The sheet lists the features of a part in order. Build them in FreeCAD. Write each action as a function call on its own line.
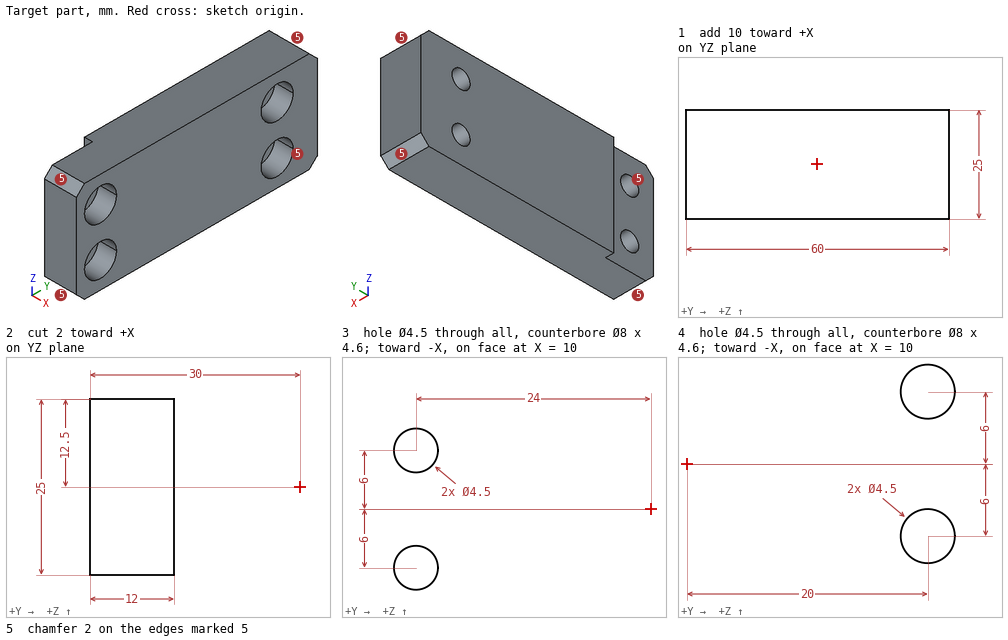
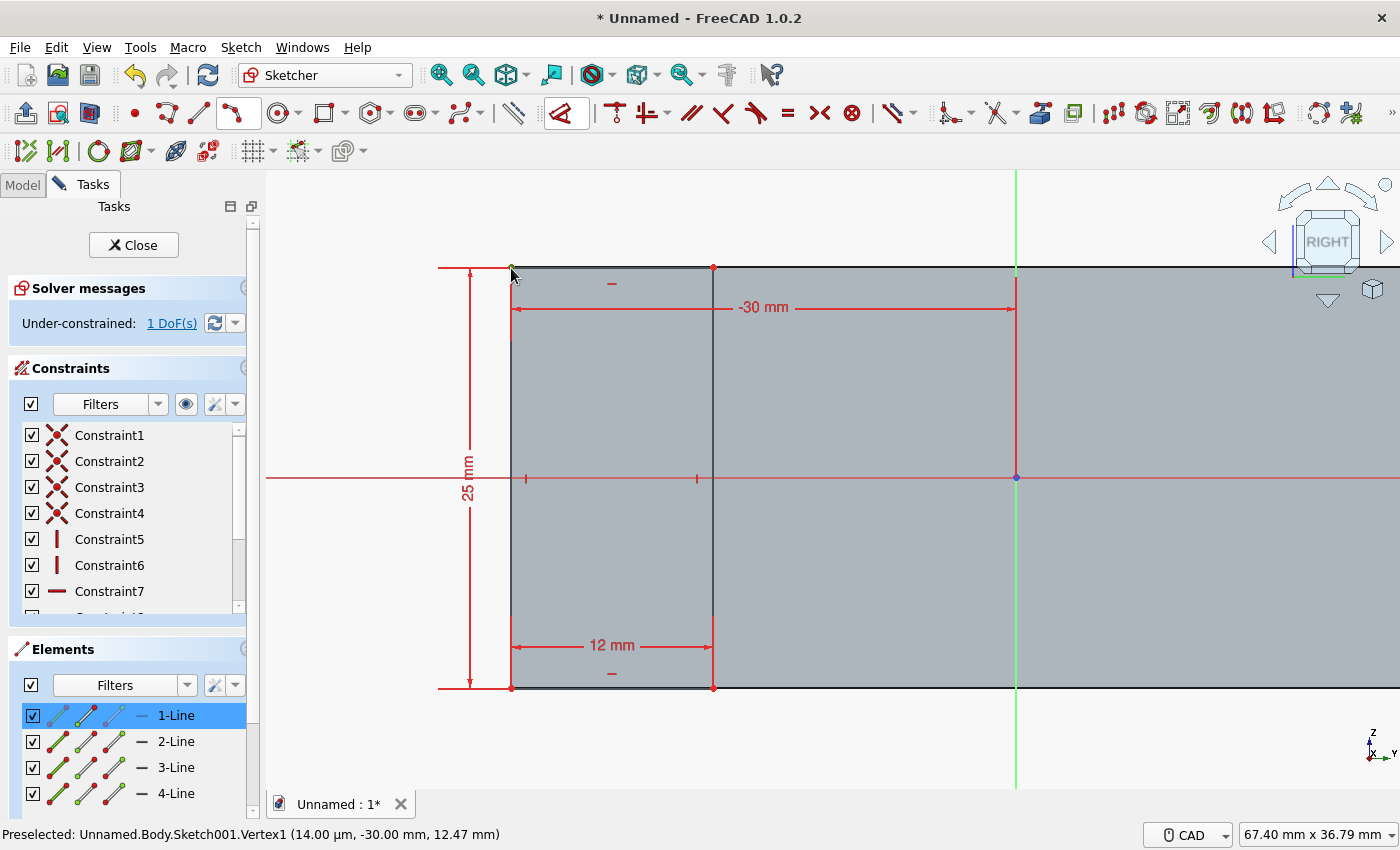
key(i)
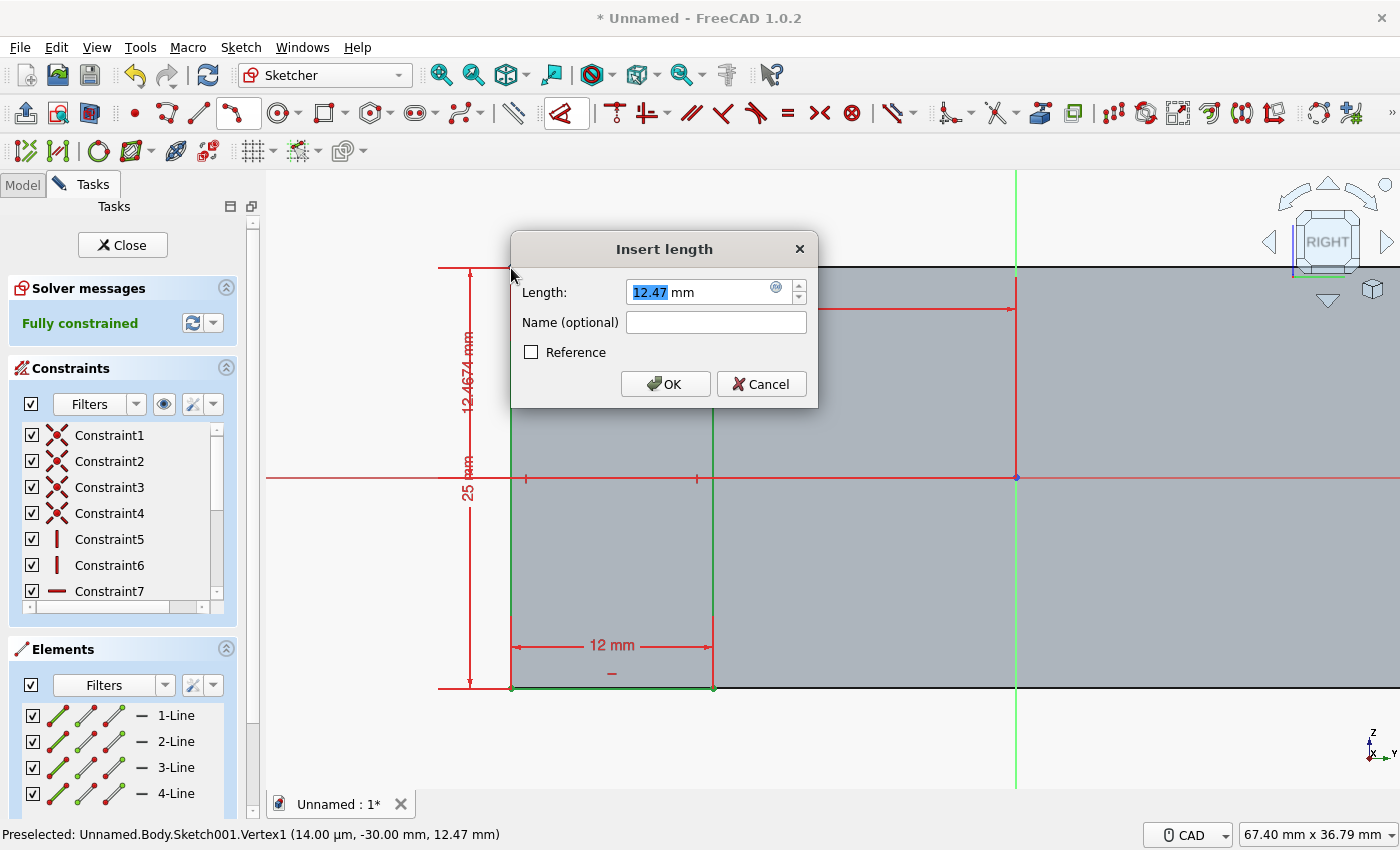
text(12.5)
key(Return)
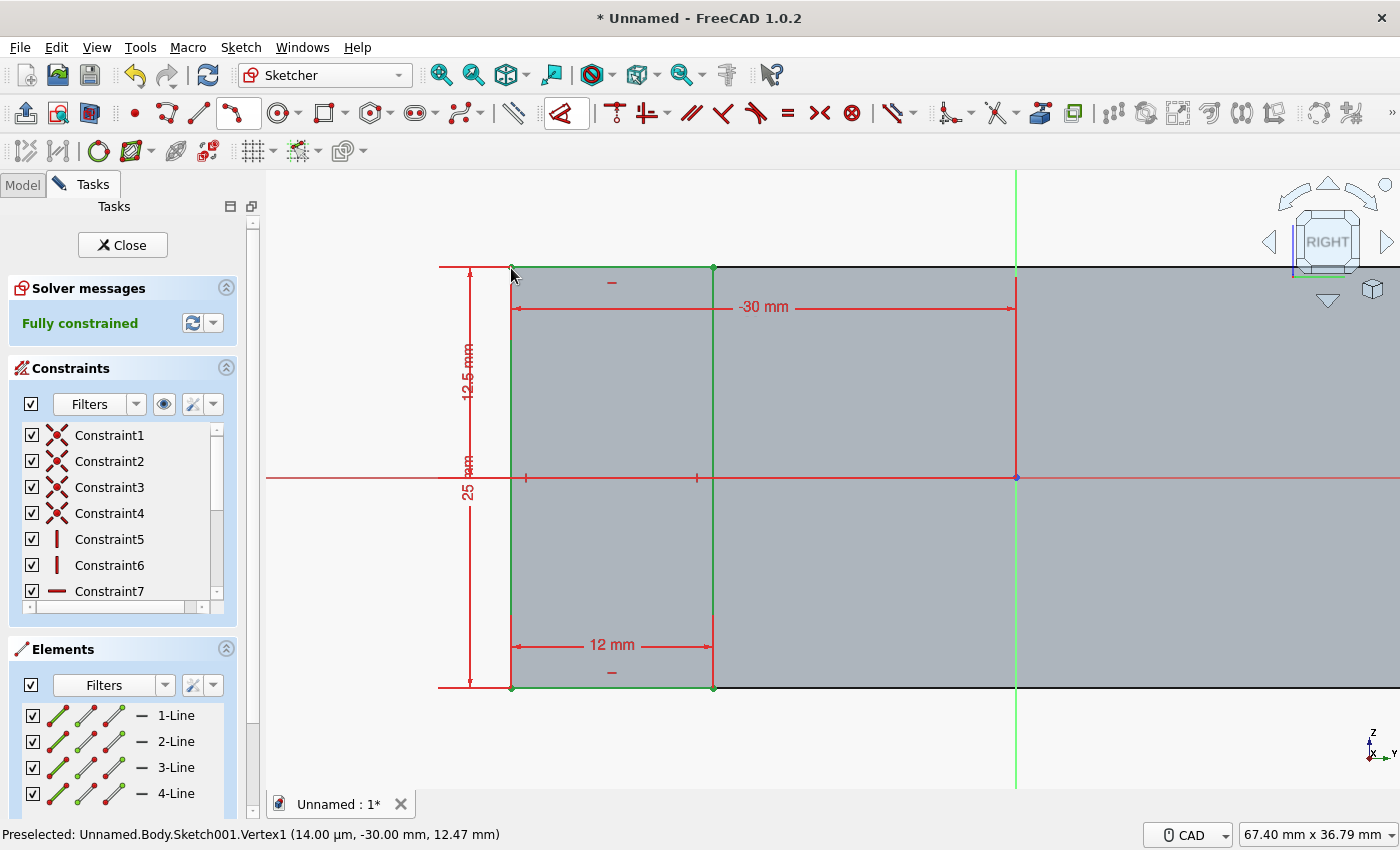
click(123, 245)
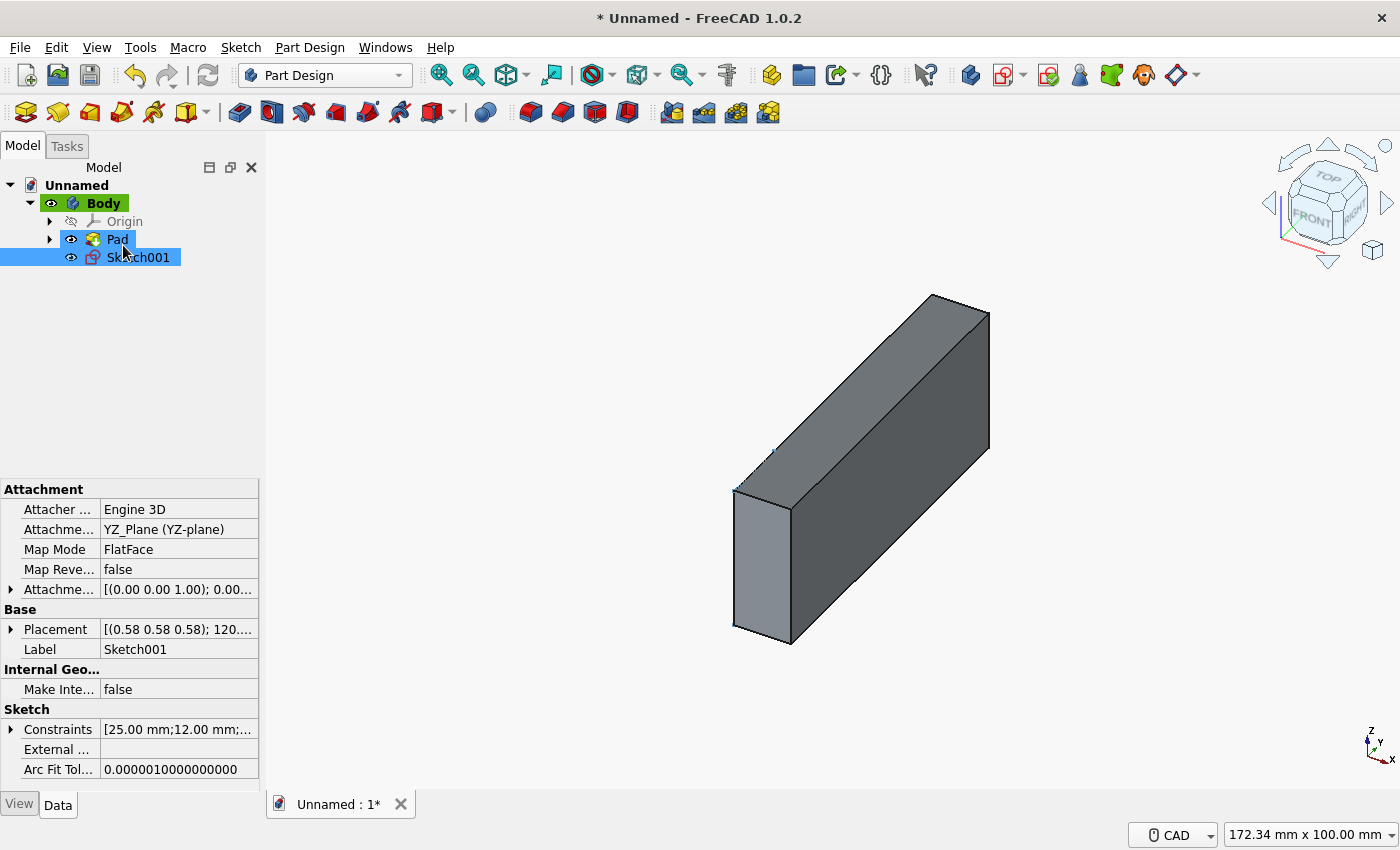
click(240, 112)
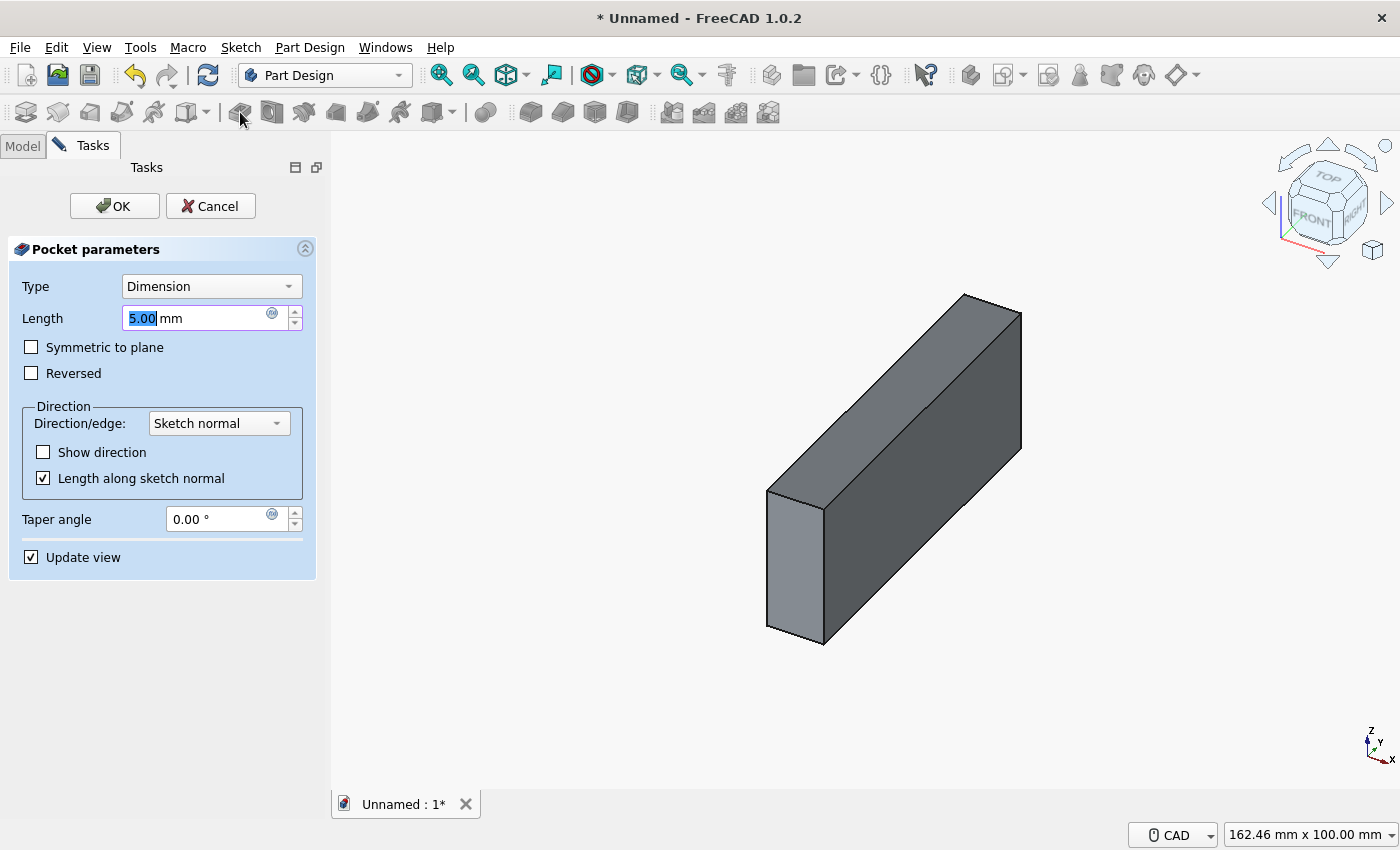
text(2)
key(Tab)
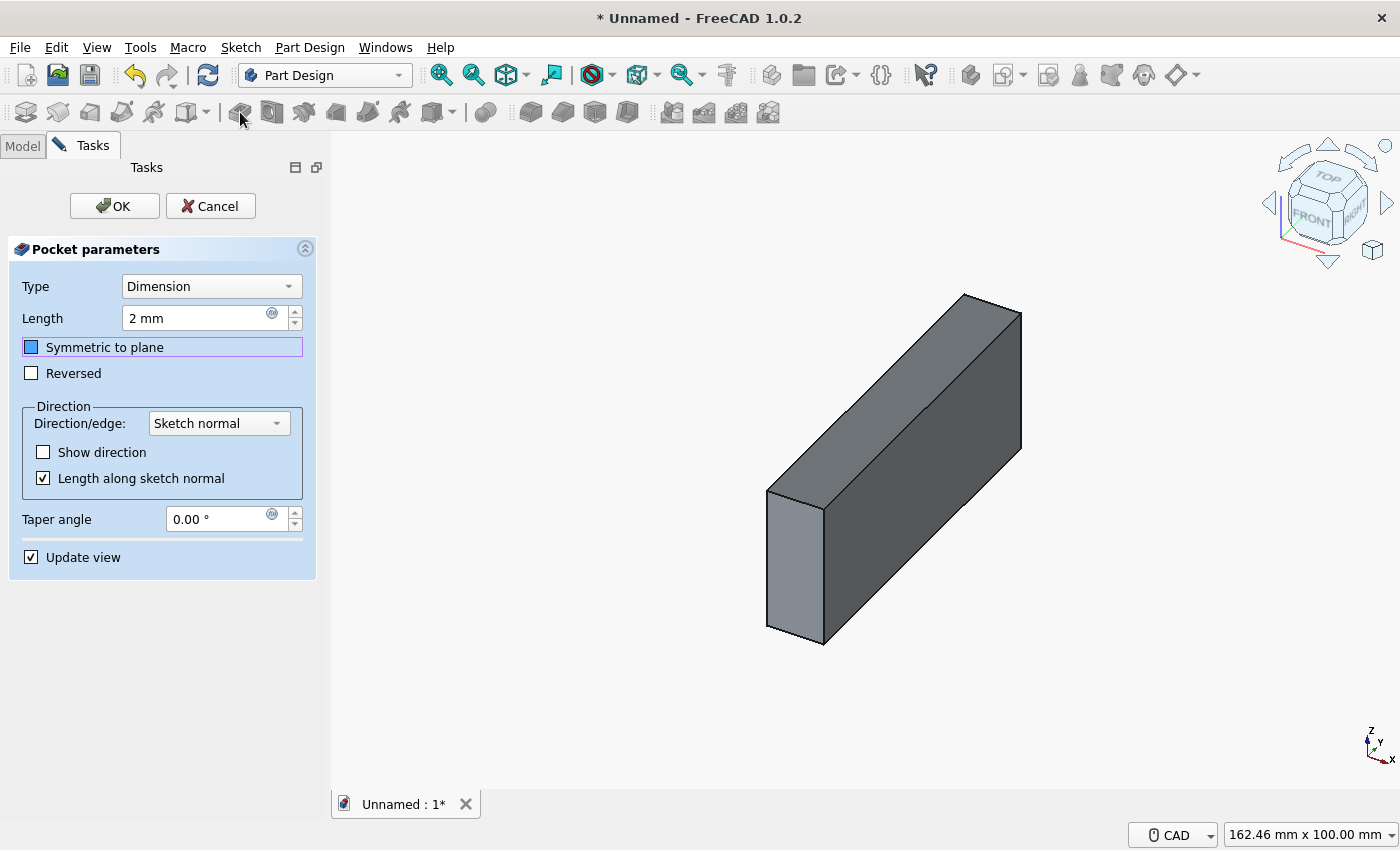
click(30, 373)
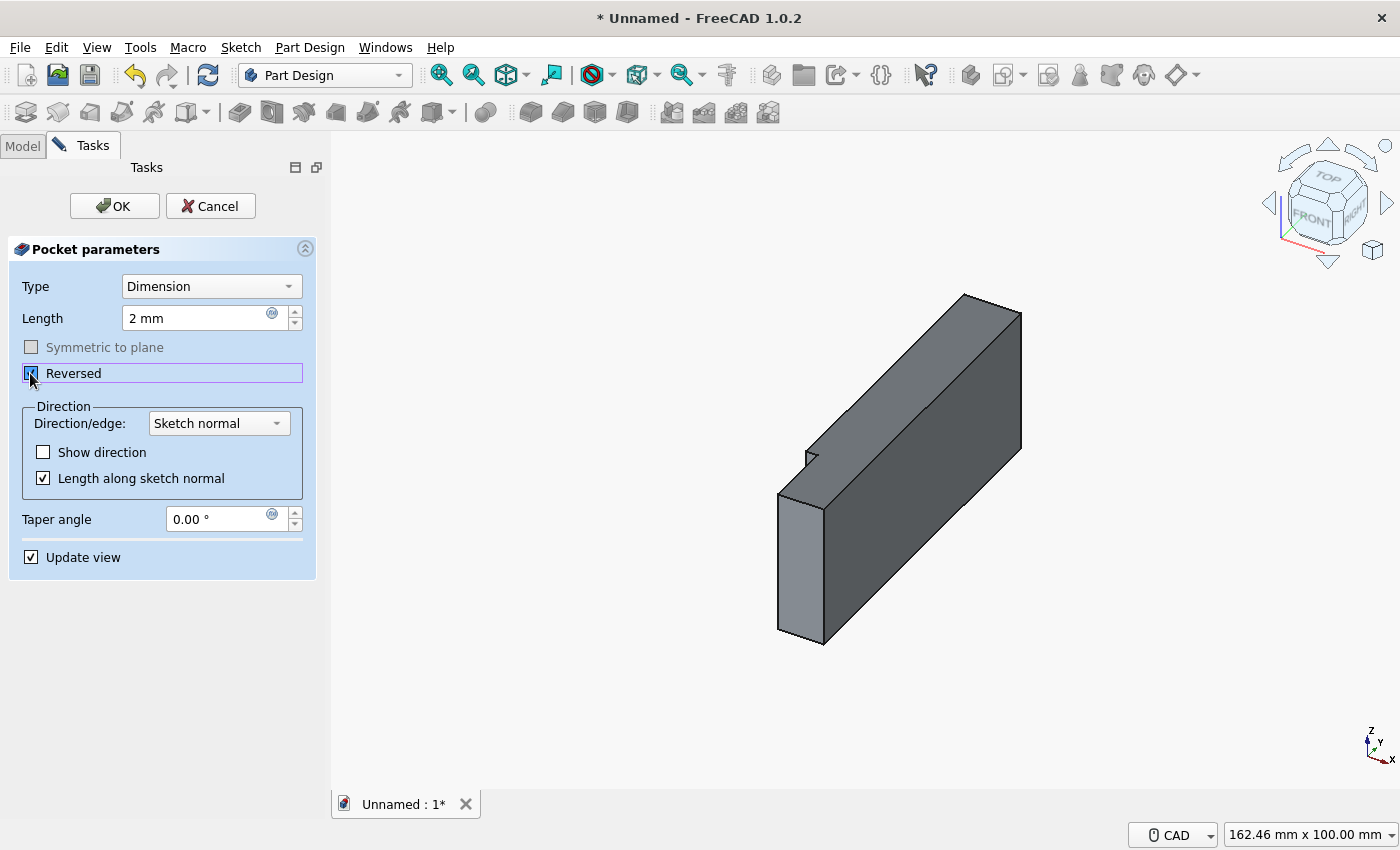
click(115, 206)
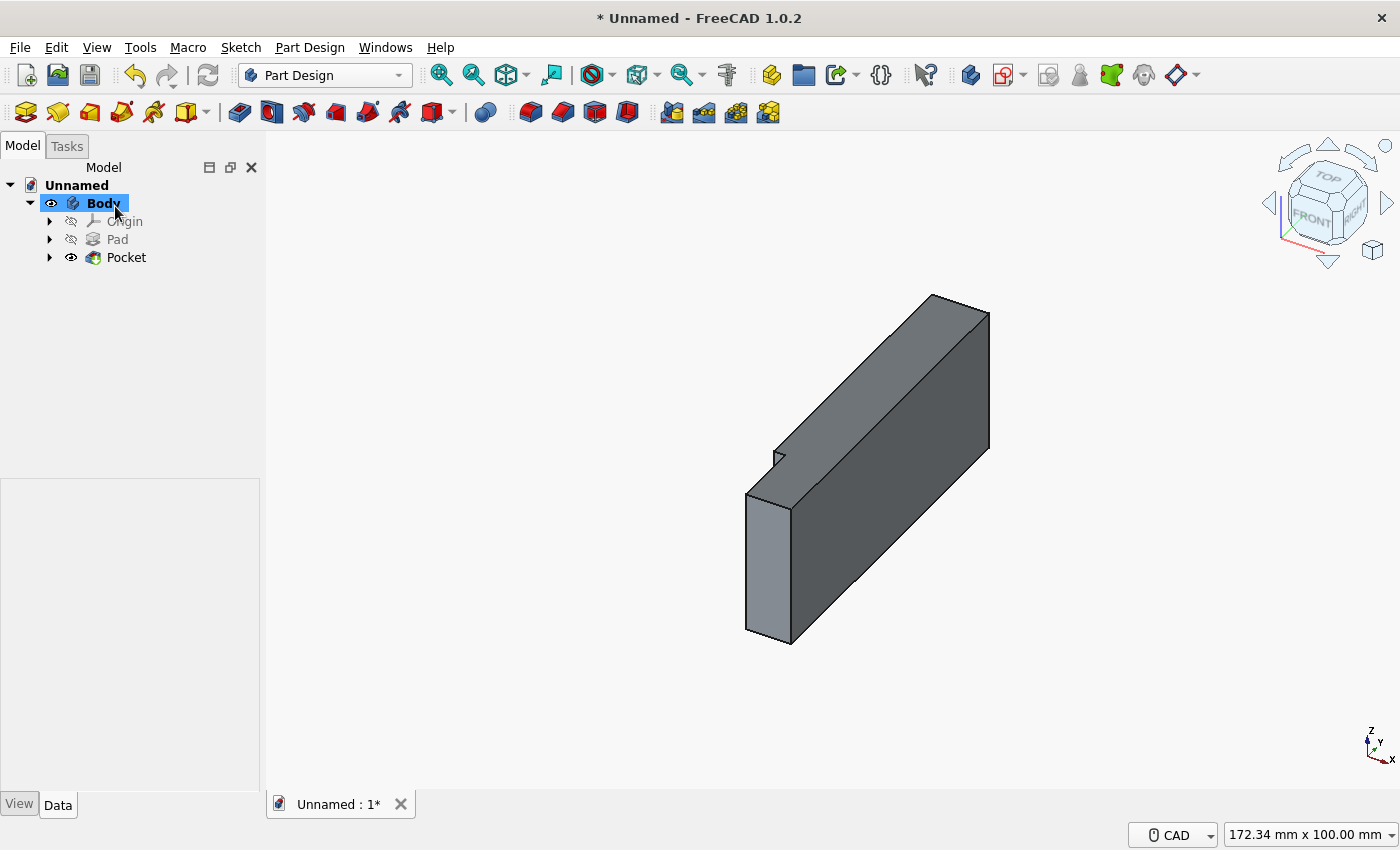
click(946, 422)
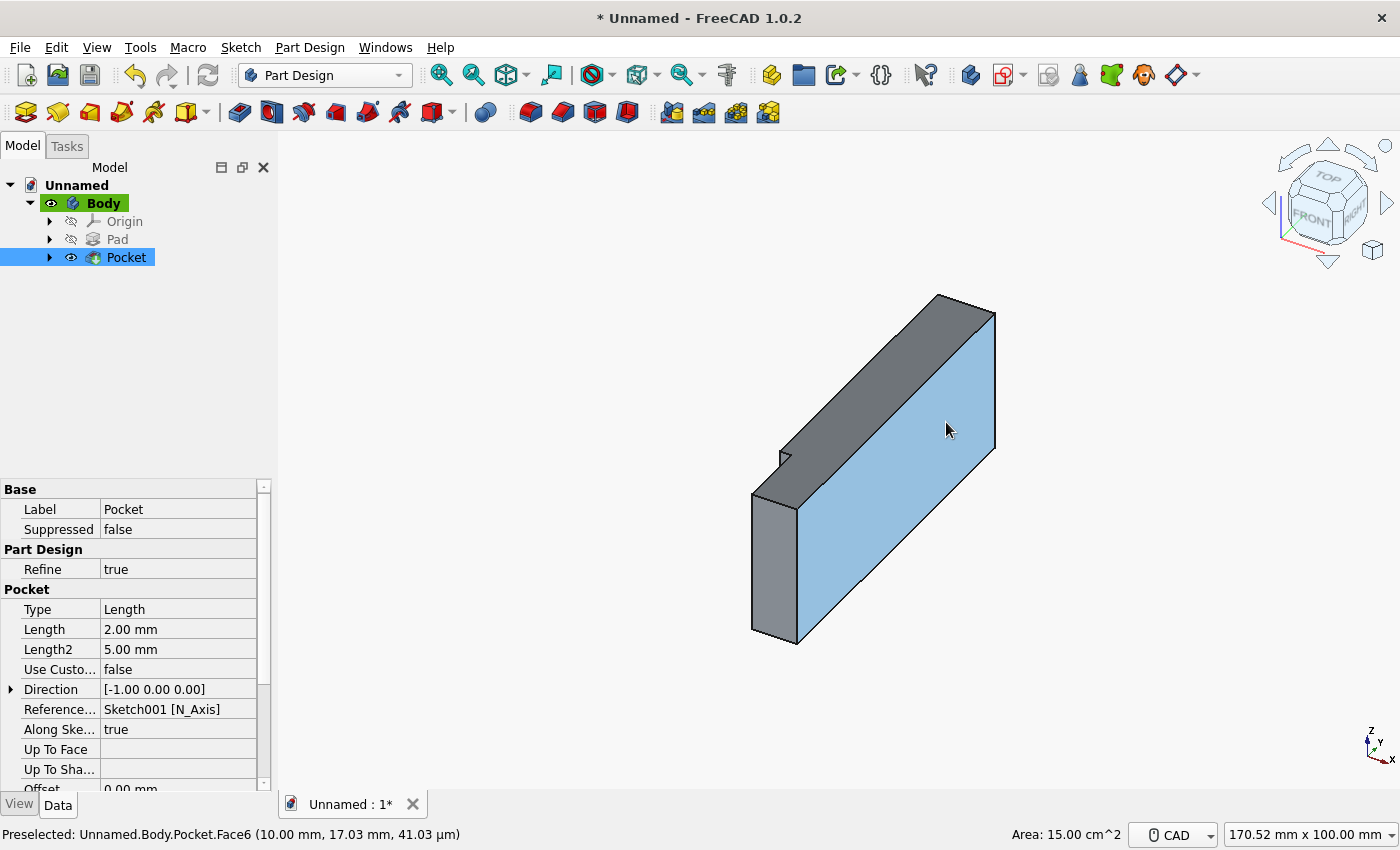
click(1004, 76)